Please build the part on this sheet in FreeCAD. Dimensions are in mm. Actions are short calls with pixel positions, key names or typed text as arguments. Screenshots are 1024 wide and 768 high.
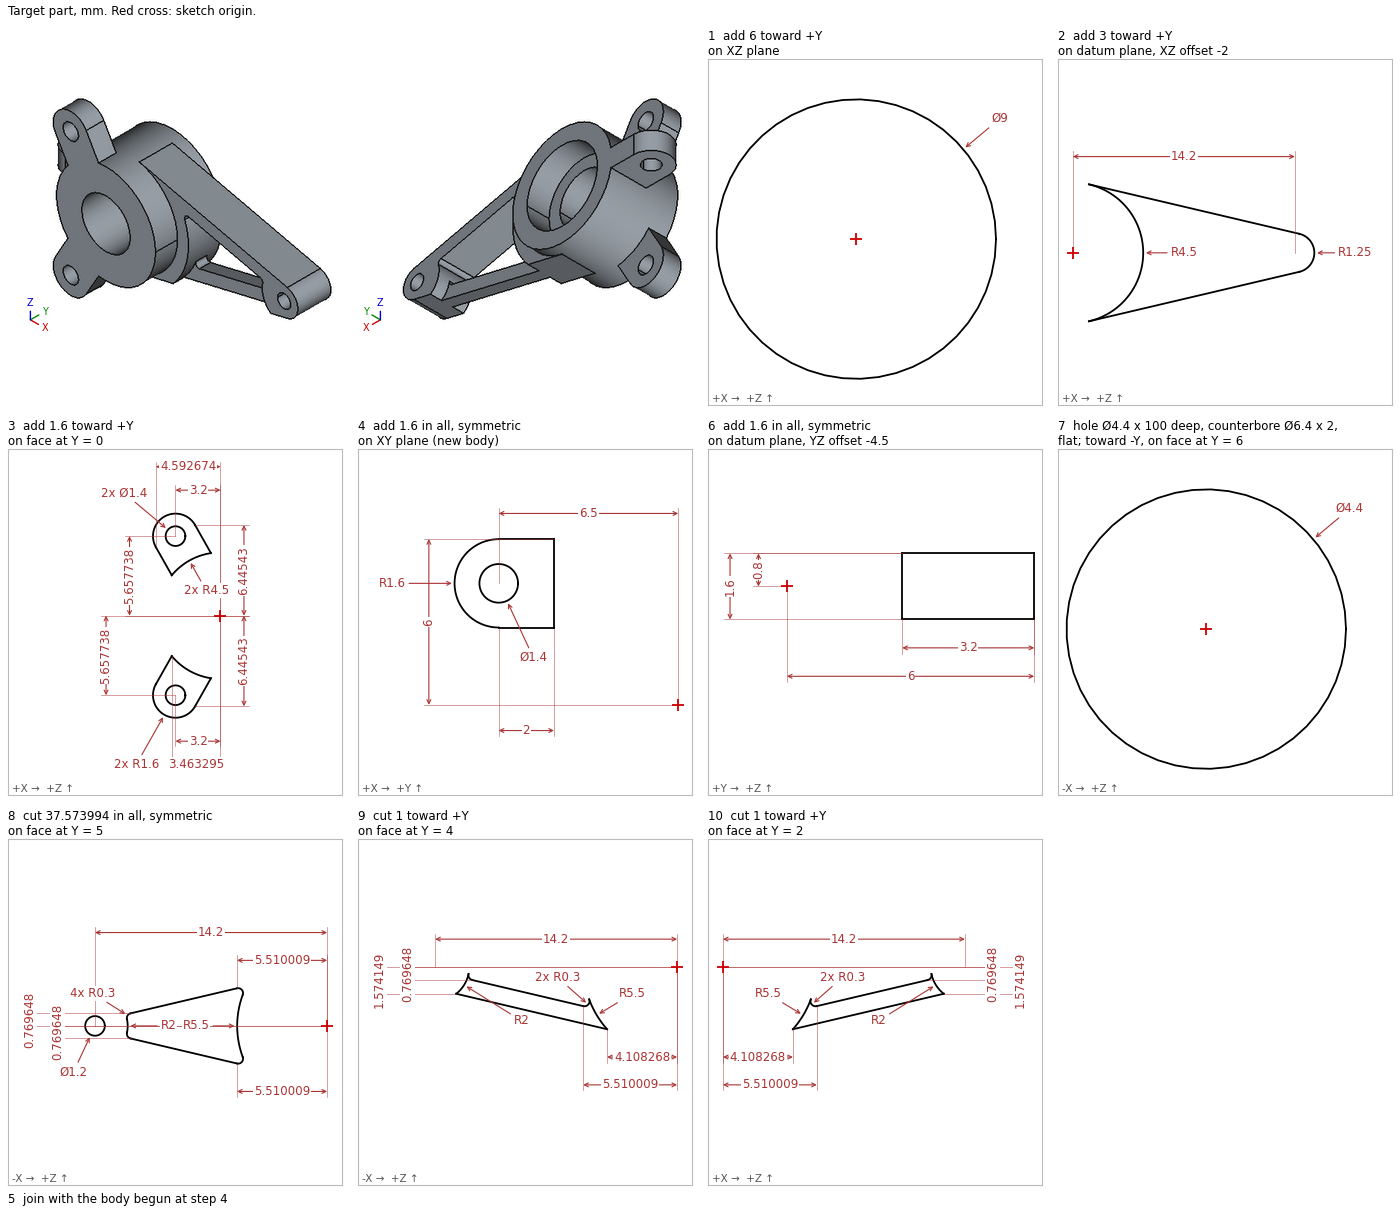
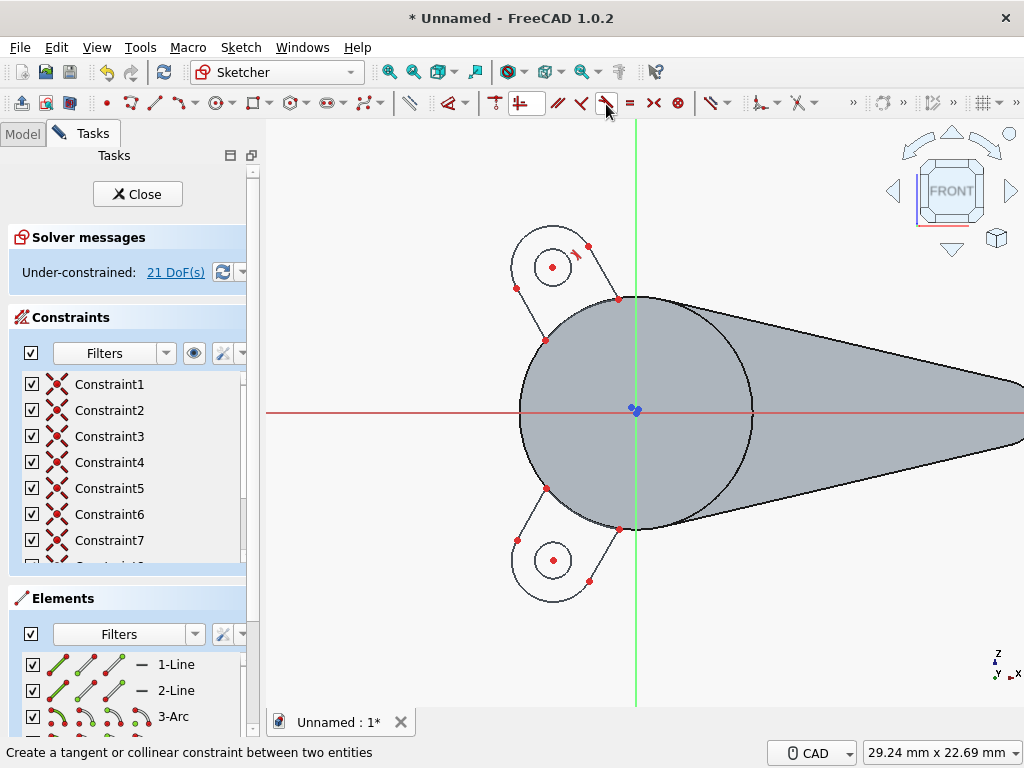
click(526, 304)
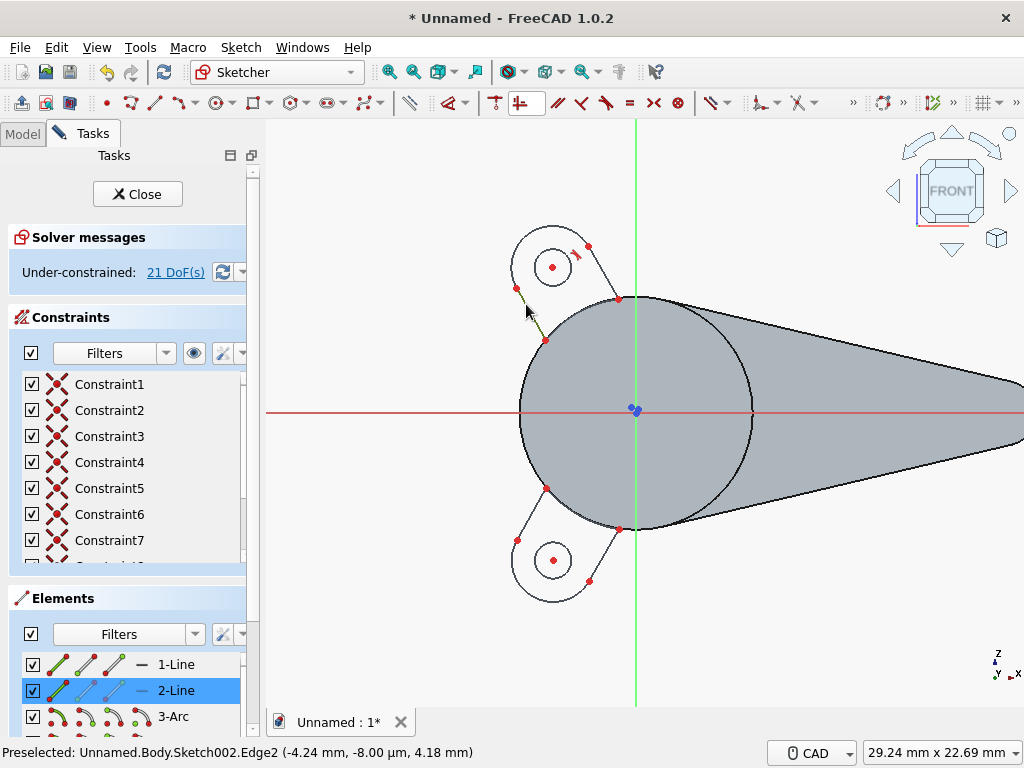
click(557, 226)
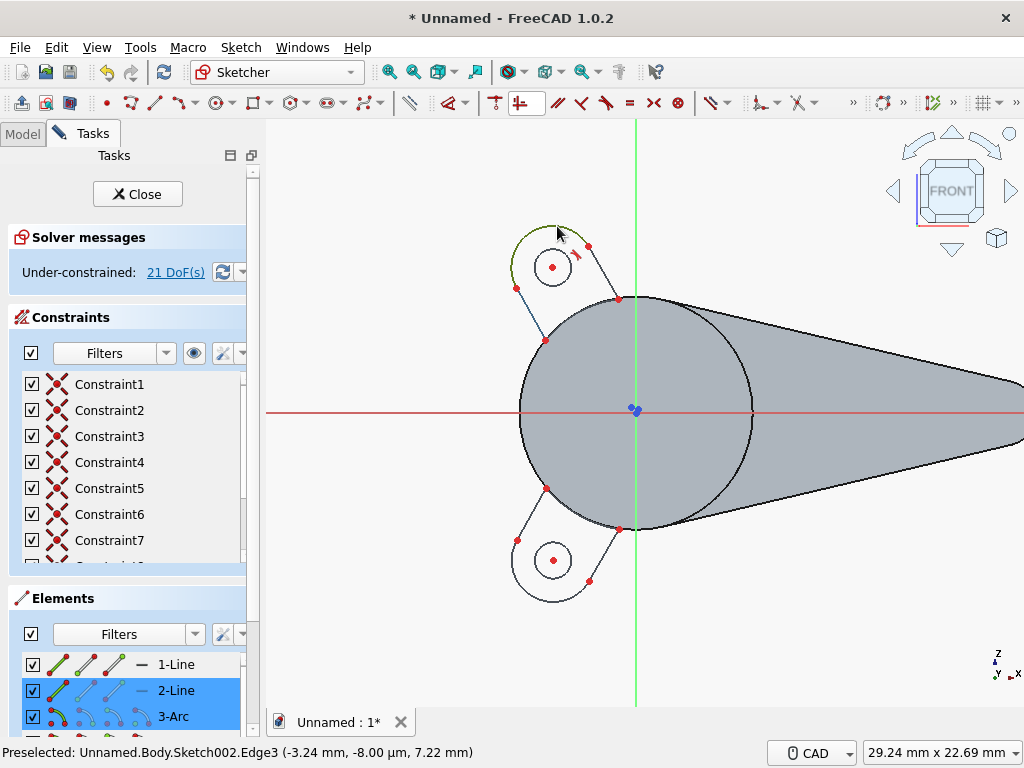
click(606, 104)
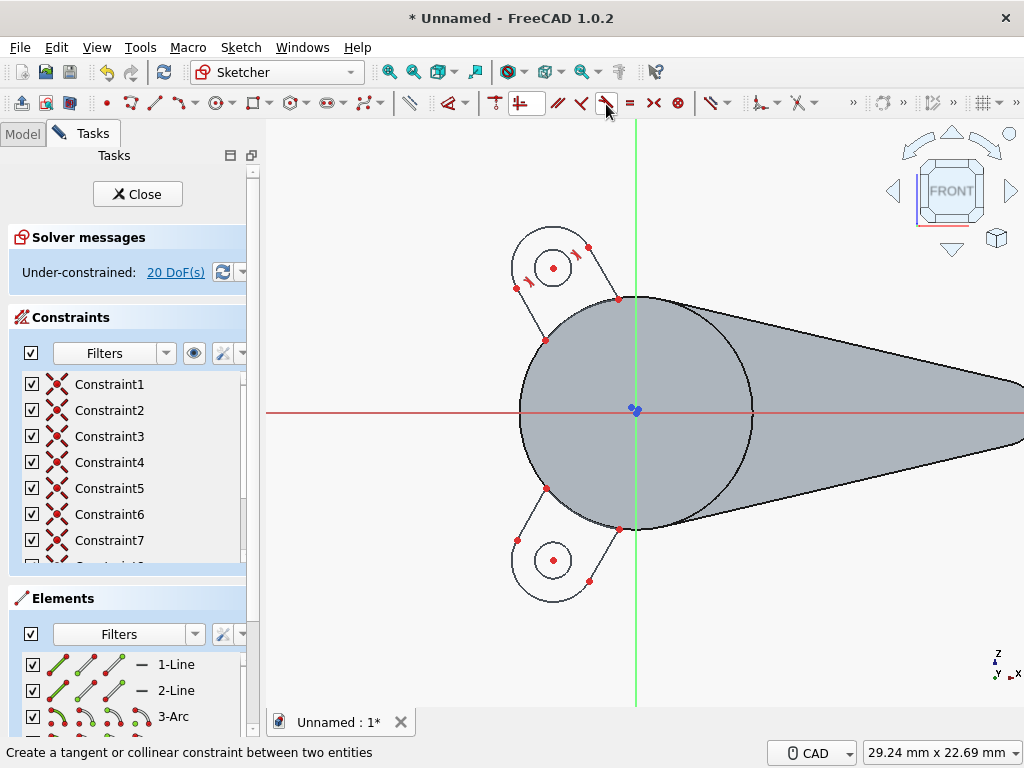
click(598, 566)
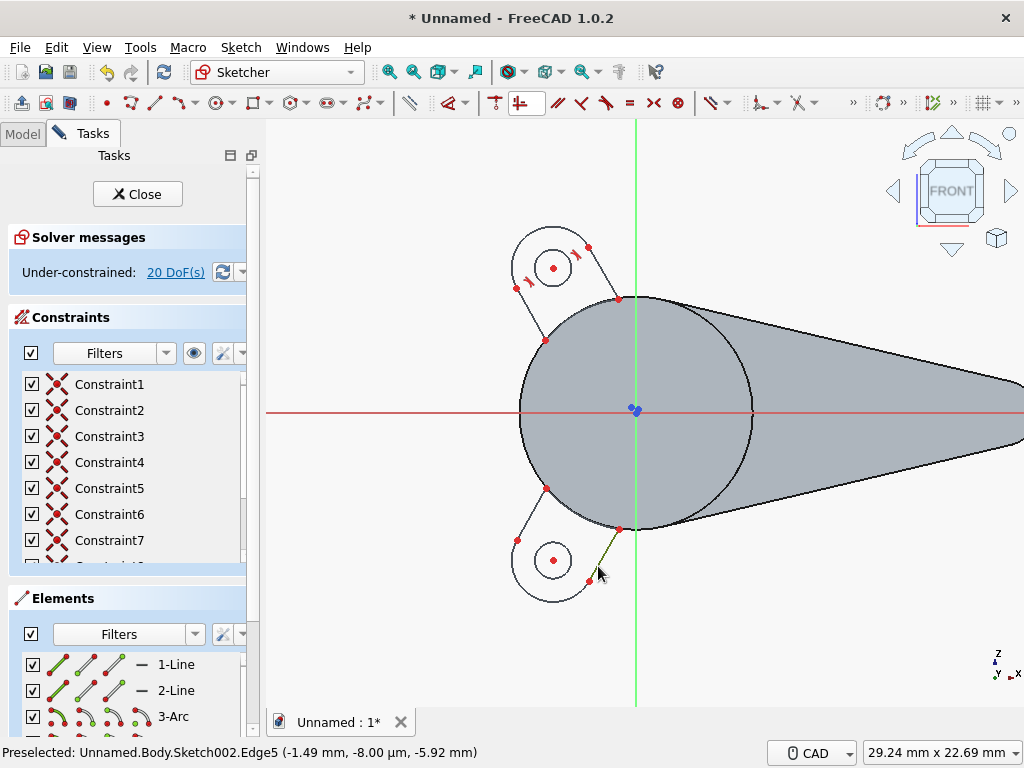
click(515, 578)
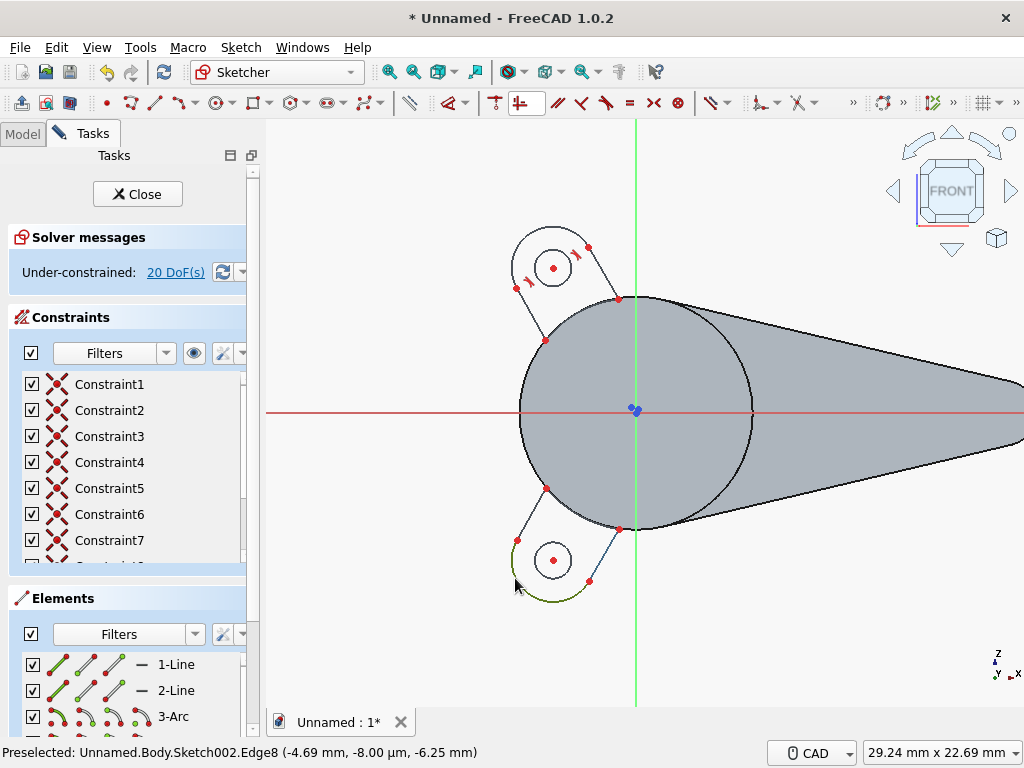
key(t)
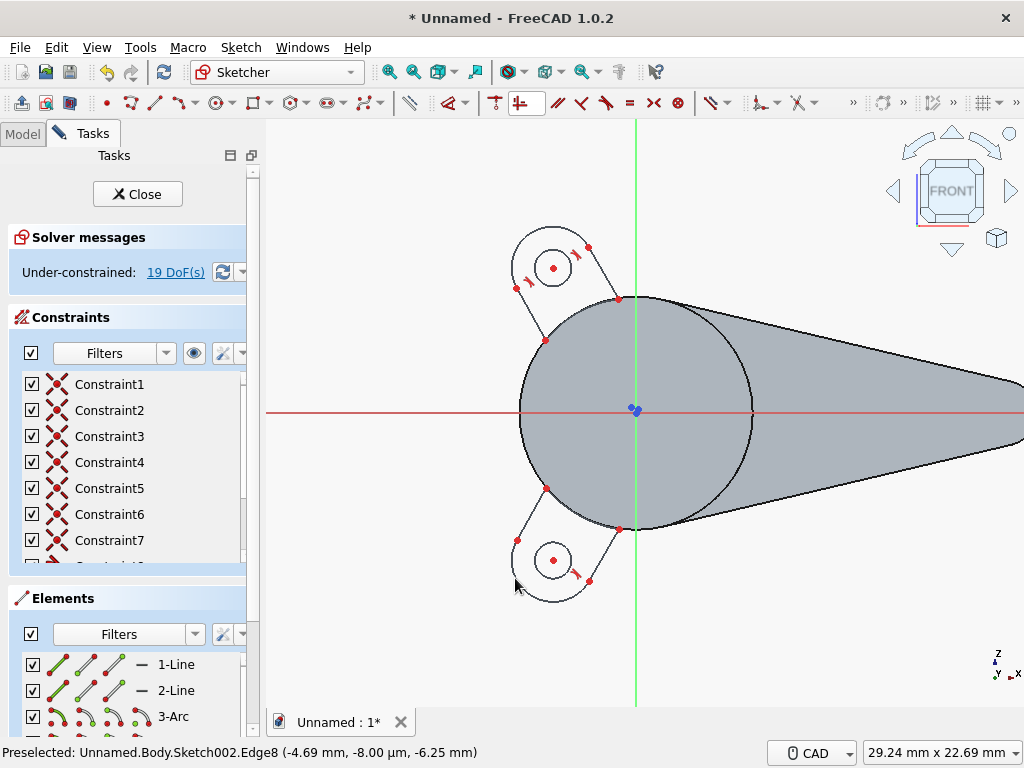
click(537, 504)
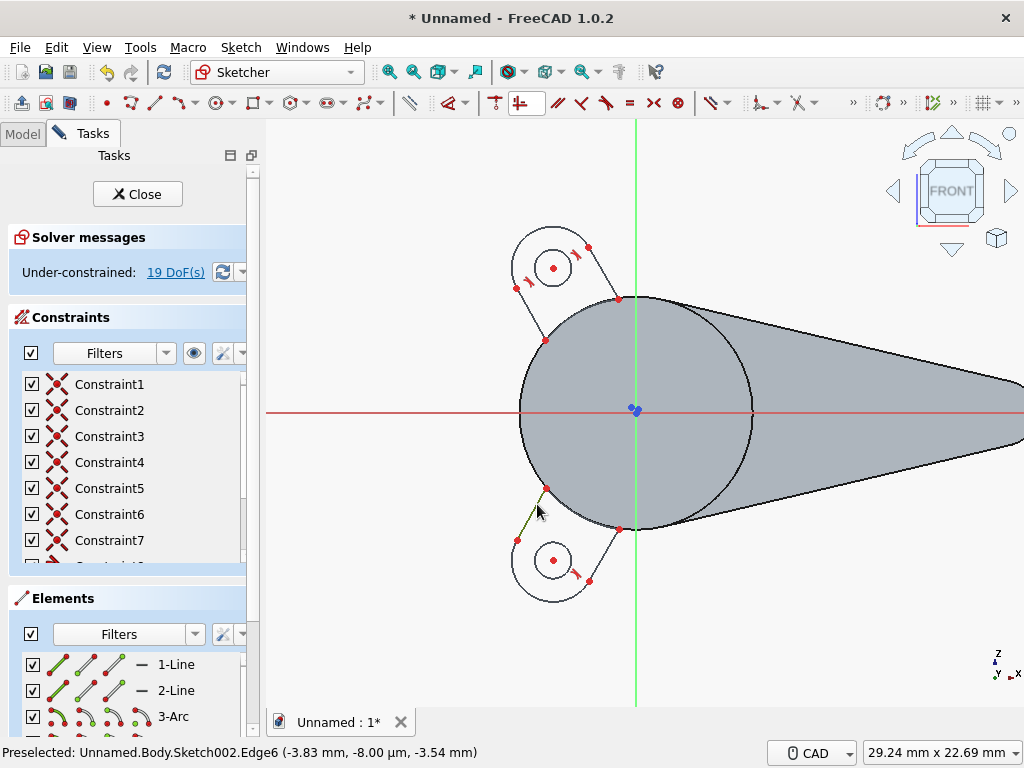
click(515, 578)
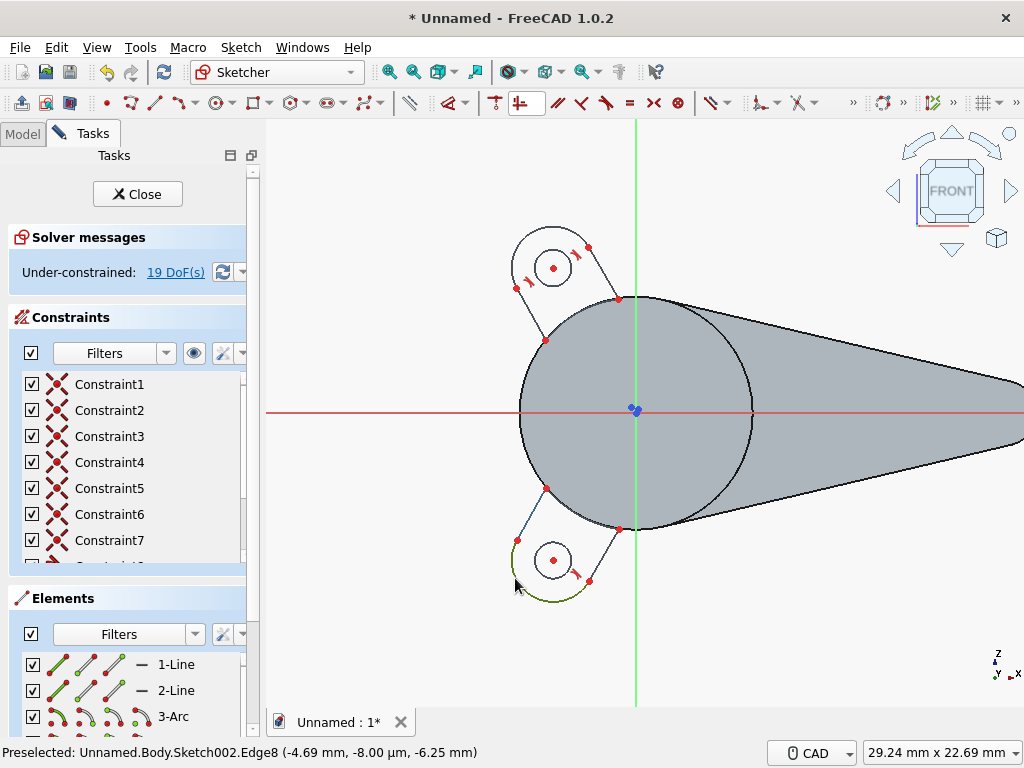
key(t)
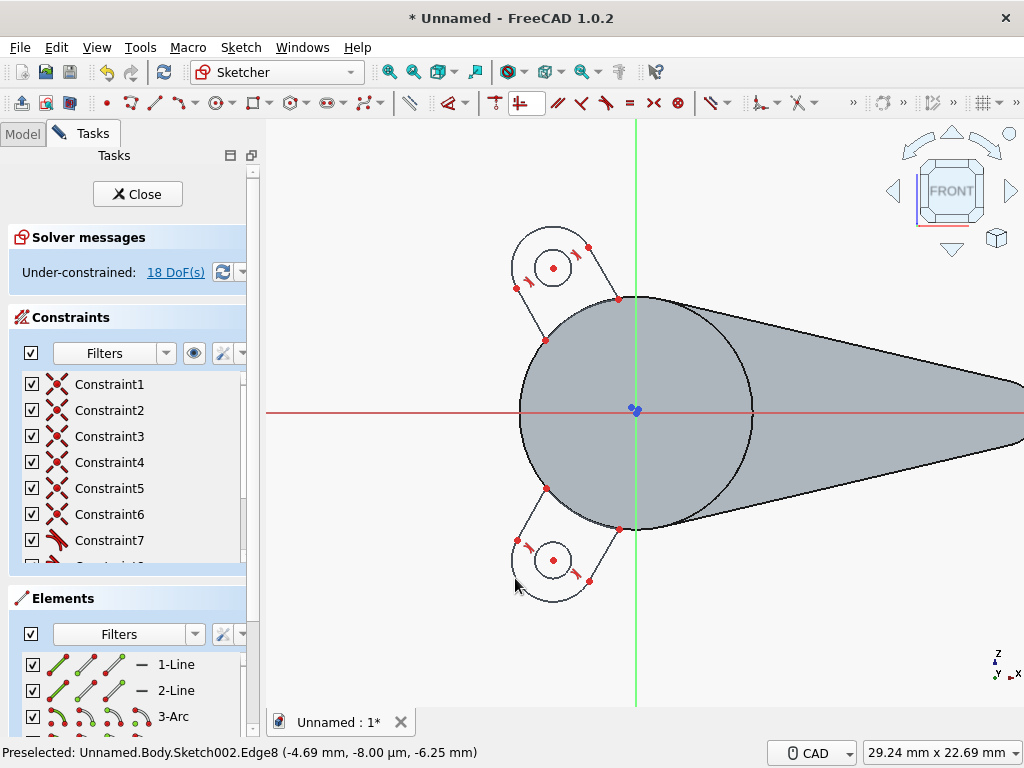
click(594, 305)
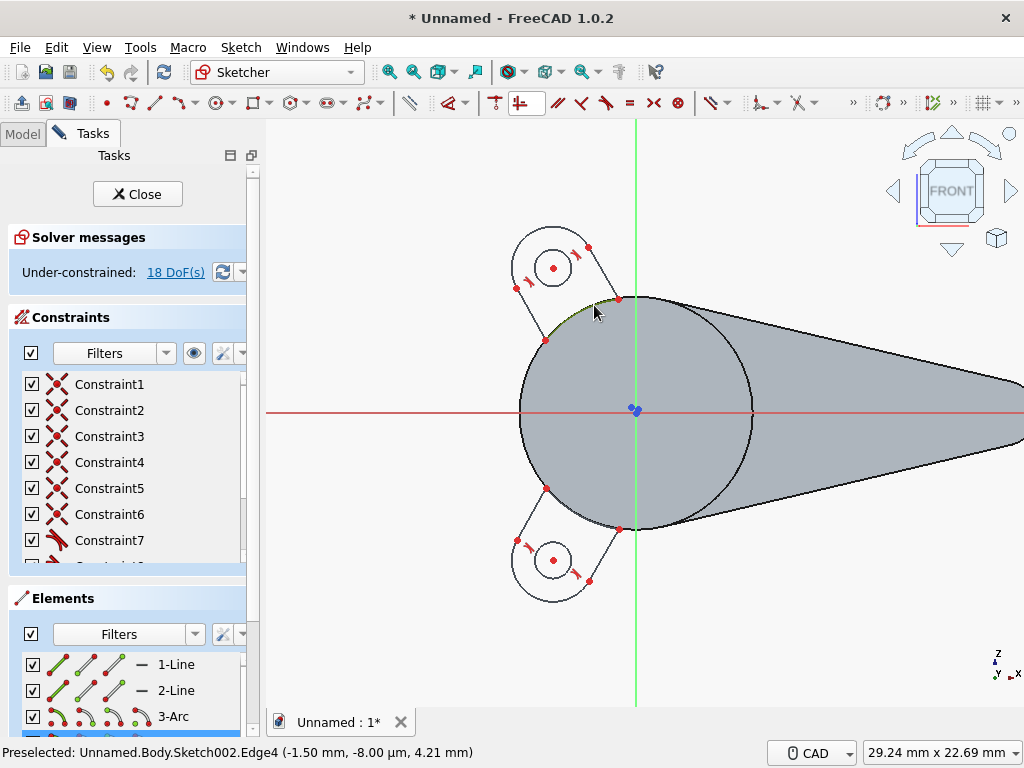
click(565, 506)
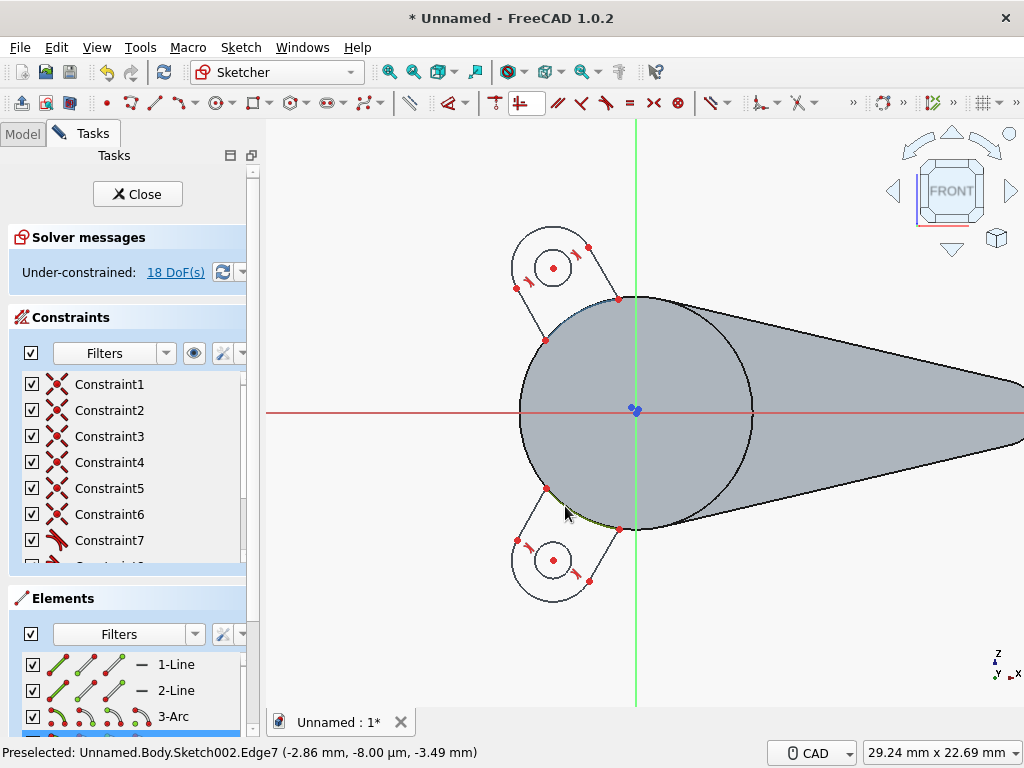
key(c)